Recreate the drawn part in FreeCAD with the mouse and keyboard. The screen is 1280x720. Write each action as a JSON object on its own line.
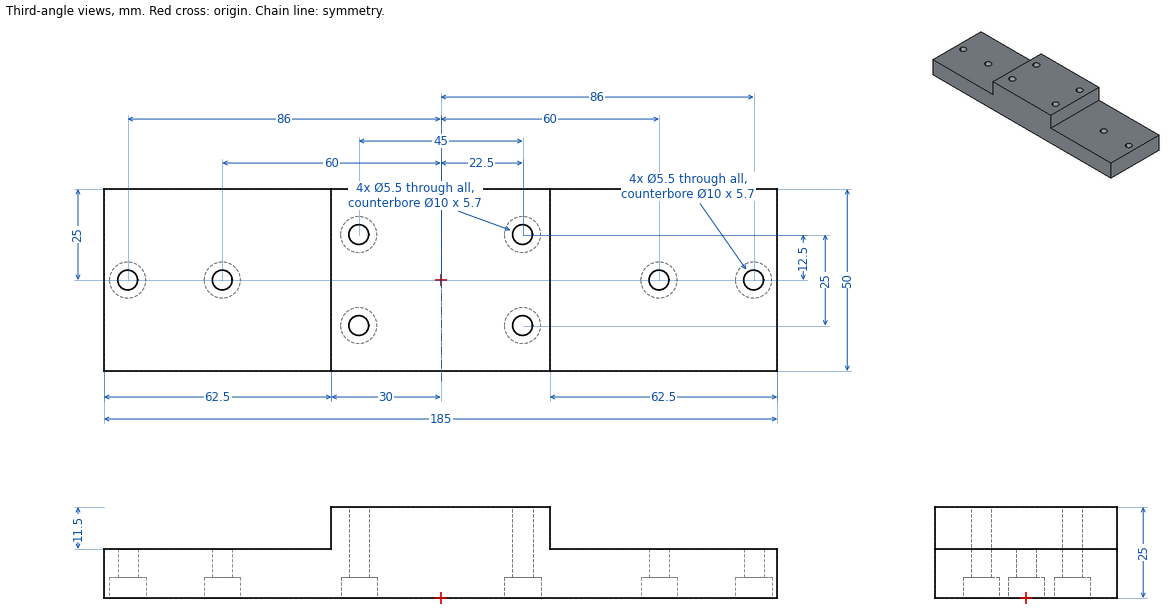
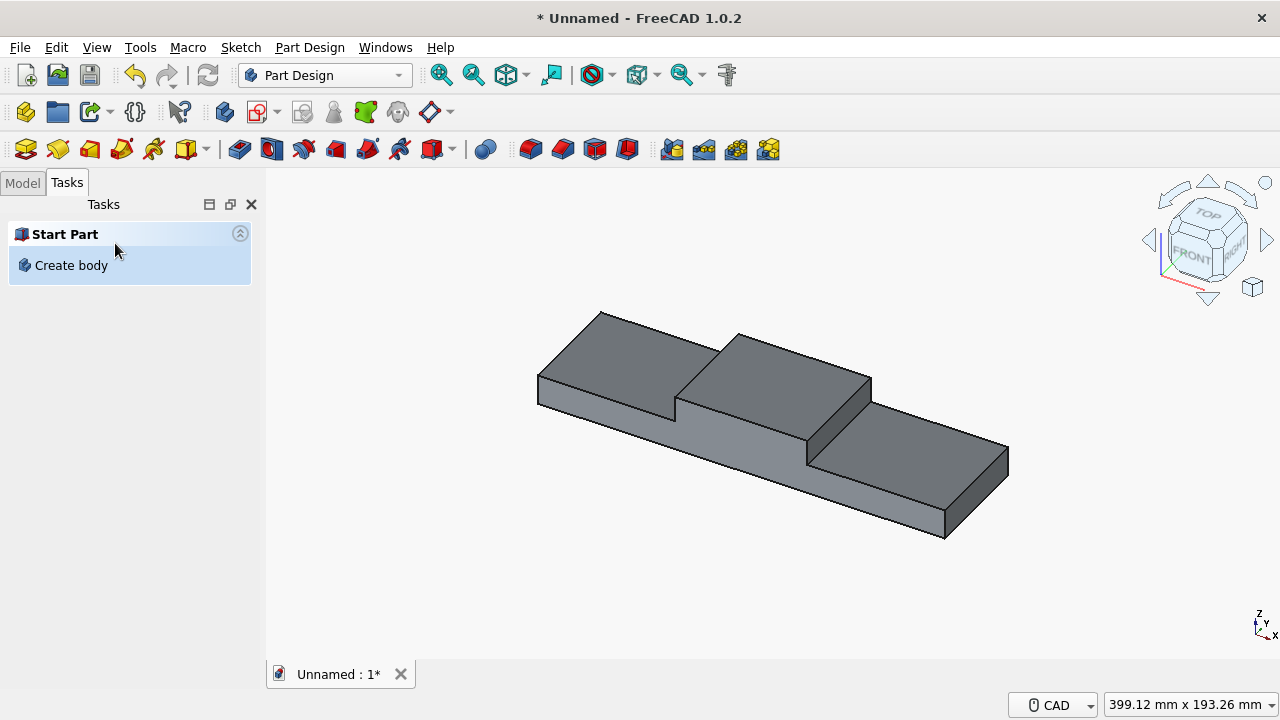
{"action": "key", "text": "5"}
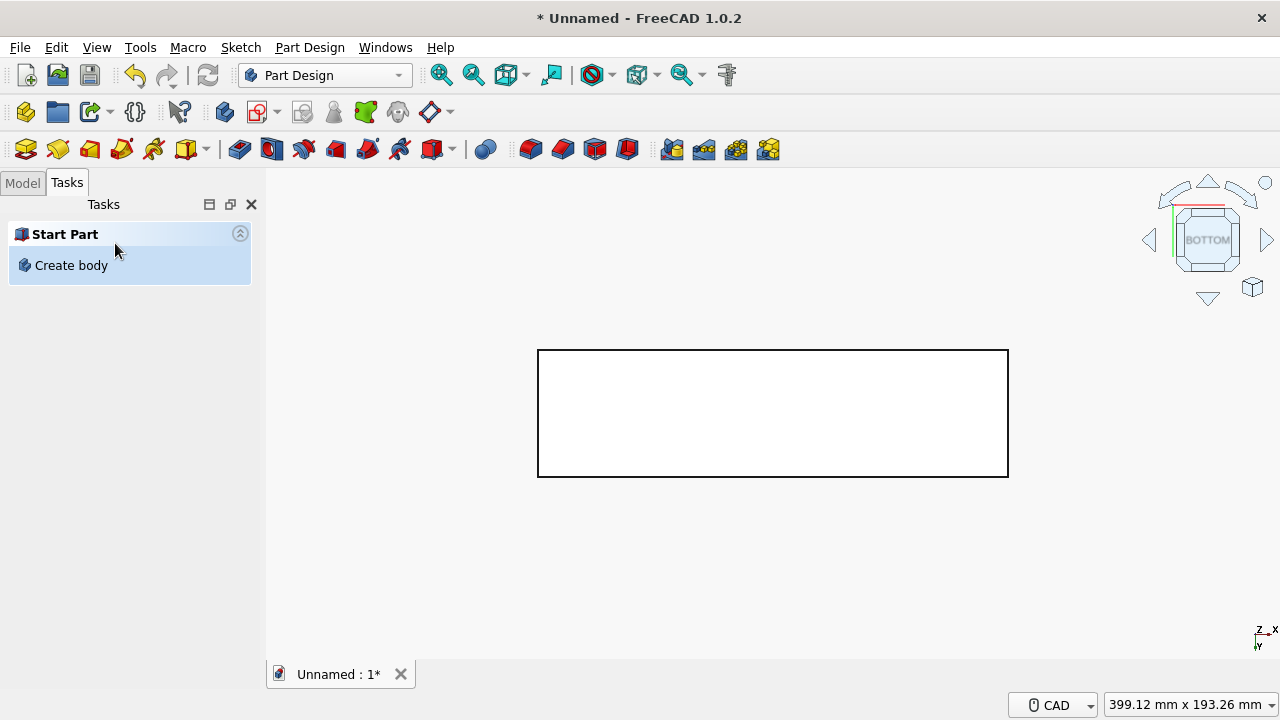
{"action": "left_click", "coordinate": [907, 412]}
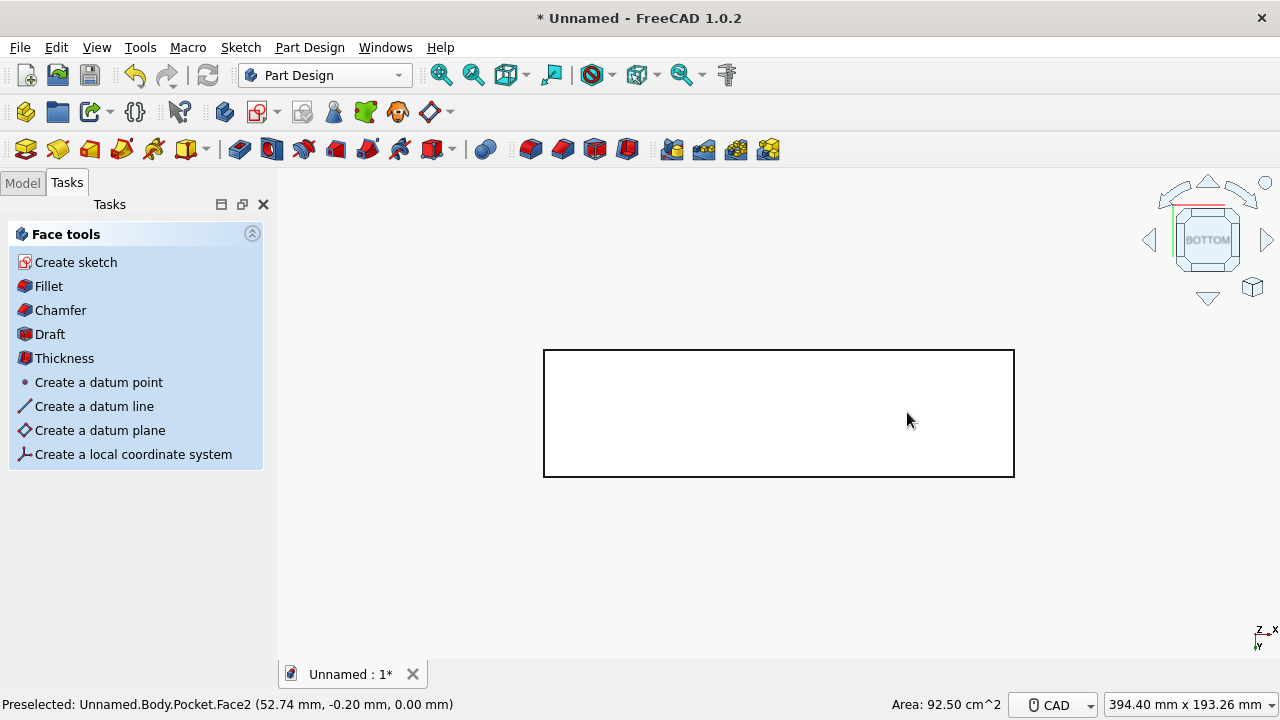
{"action": "left_click", "coordinate": [258, 112]}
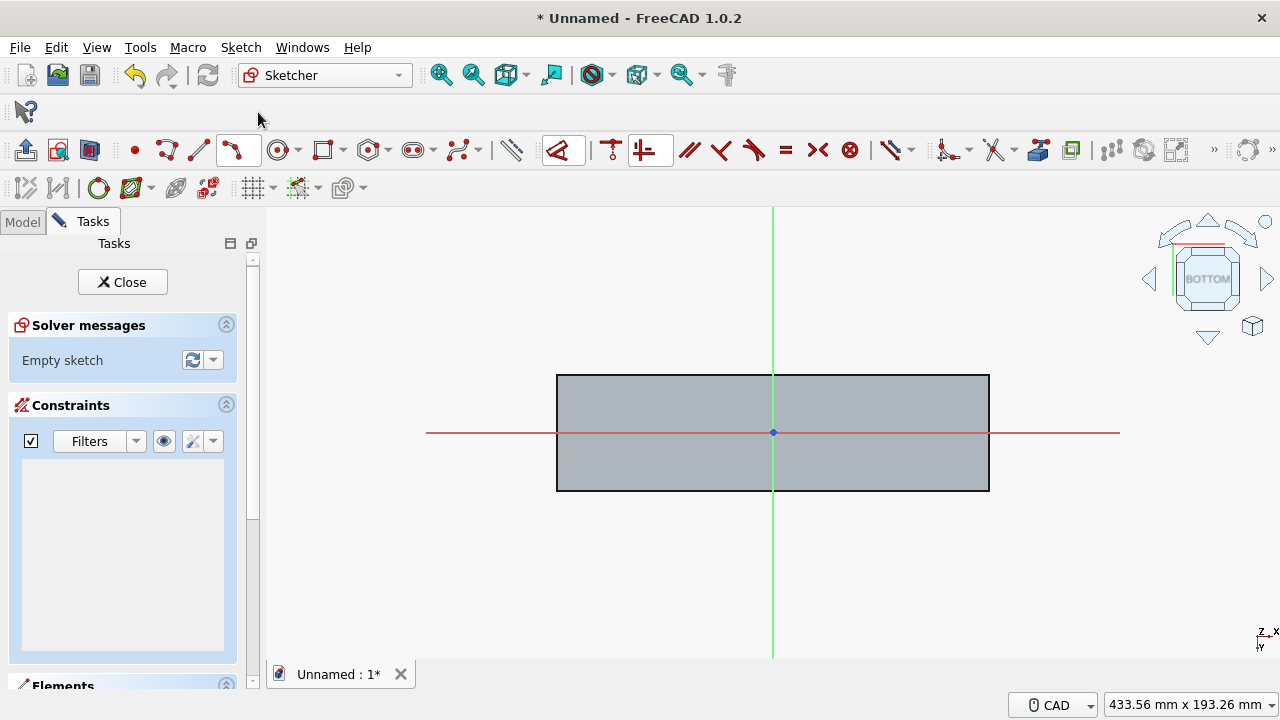
{"action": "scroll", "coordinate": [912, 433], "scroll_direction": "up", "scroll_amount": 2}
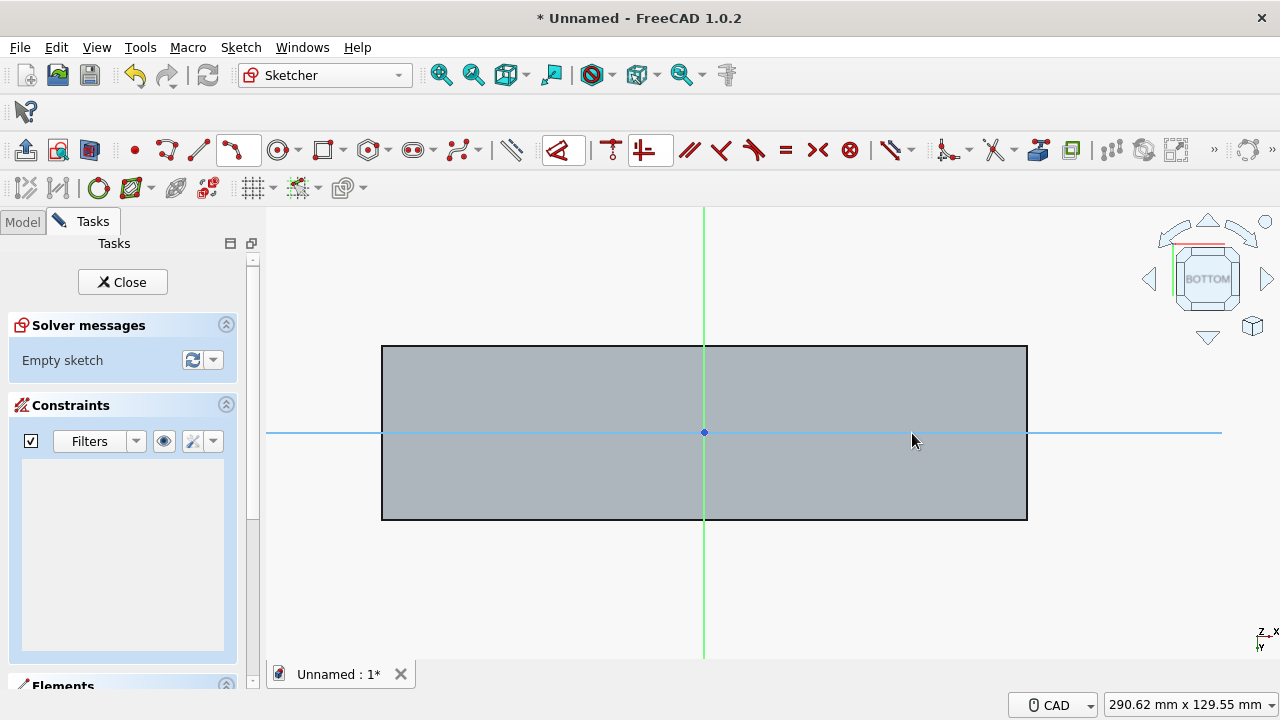
{"action": "left_click", "coordinate": [278, 150]}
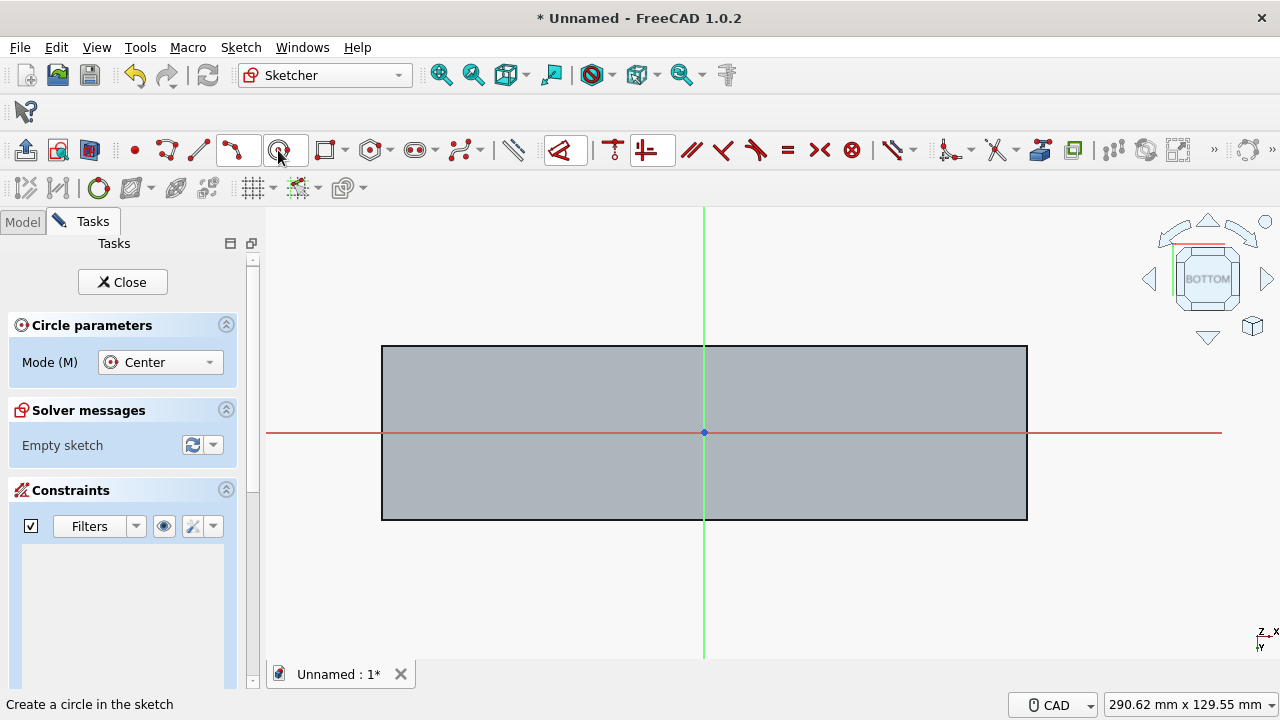
{"action": "scroll", "coordinate": [1004, 433], "scroll_direction": "up", "scroll_amount": 5}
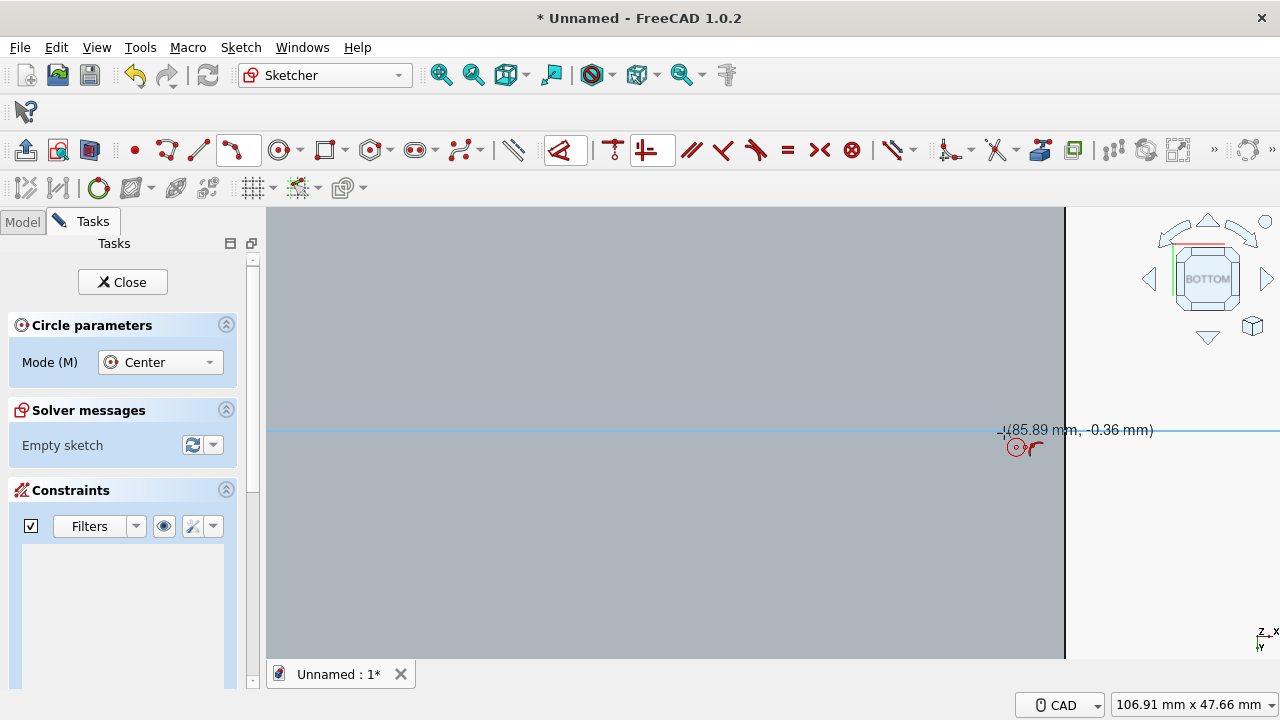
{"action": "left_click", "coordinate": [1004, 431]}
{"action": "mouse_move", "coordinate": [1022, 413]}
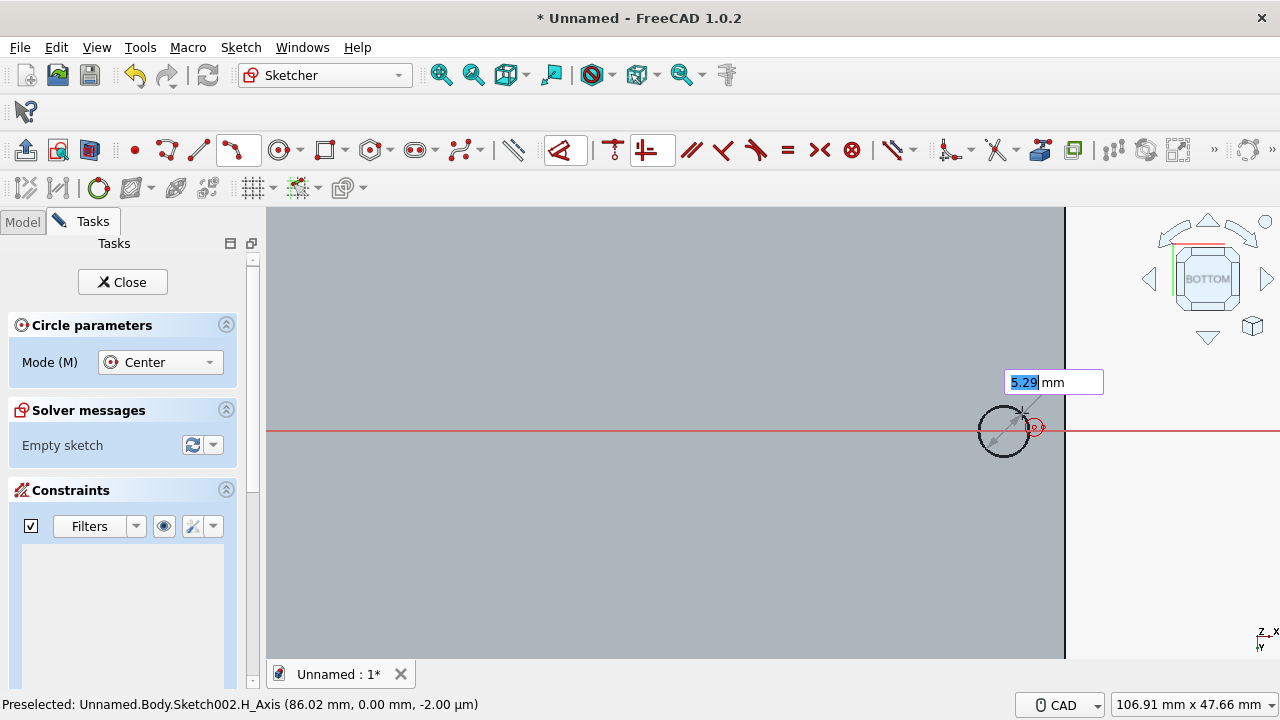
{"action": "type", "text": "5.5"}
{"action": "key", "text": "Return"}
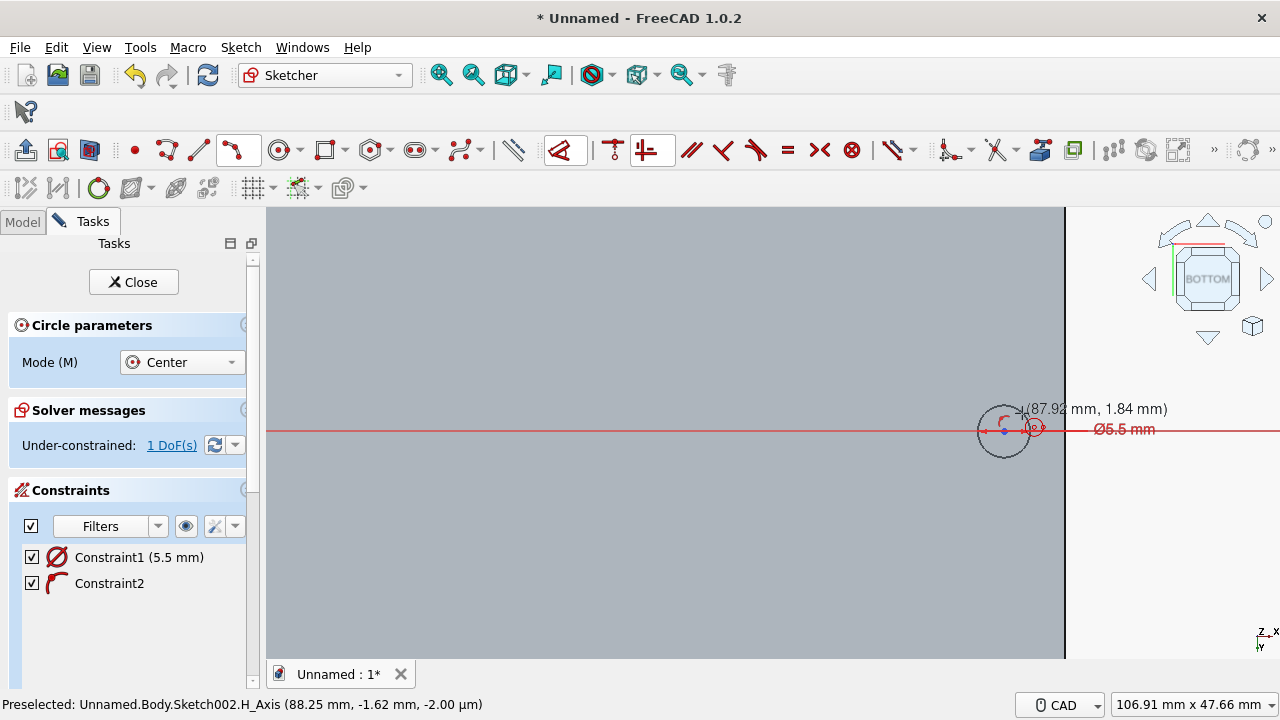
{"action": "left_click", "coordinate": [757, 431]}
{"action": "mouse_move", "coordinate": [776, 413]}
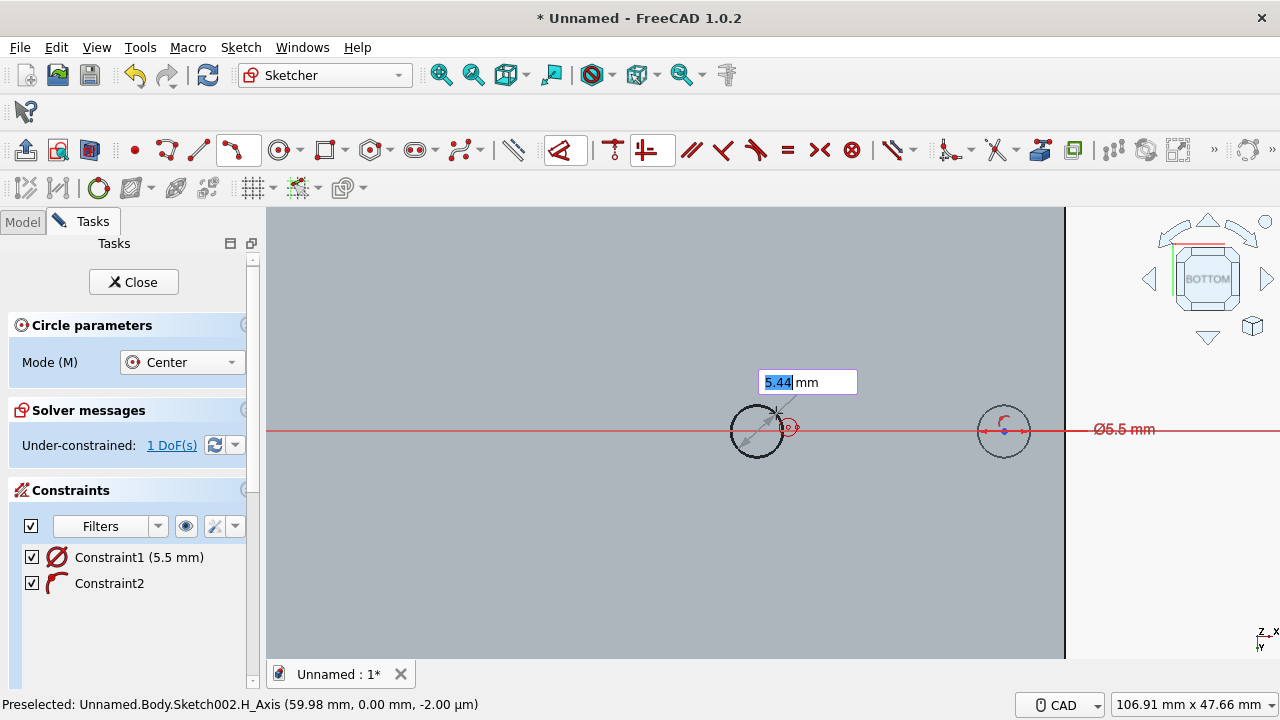
{"action": "type", "text": "5.5"}
{"action": "key", "text": "Return"}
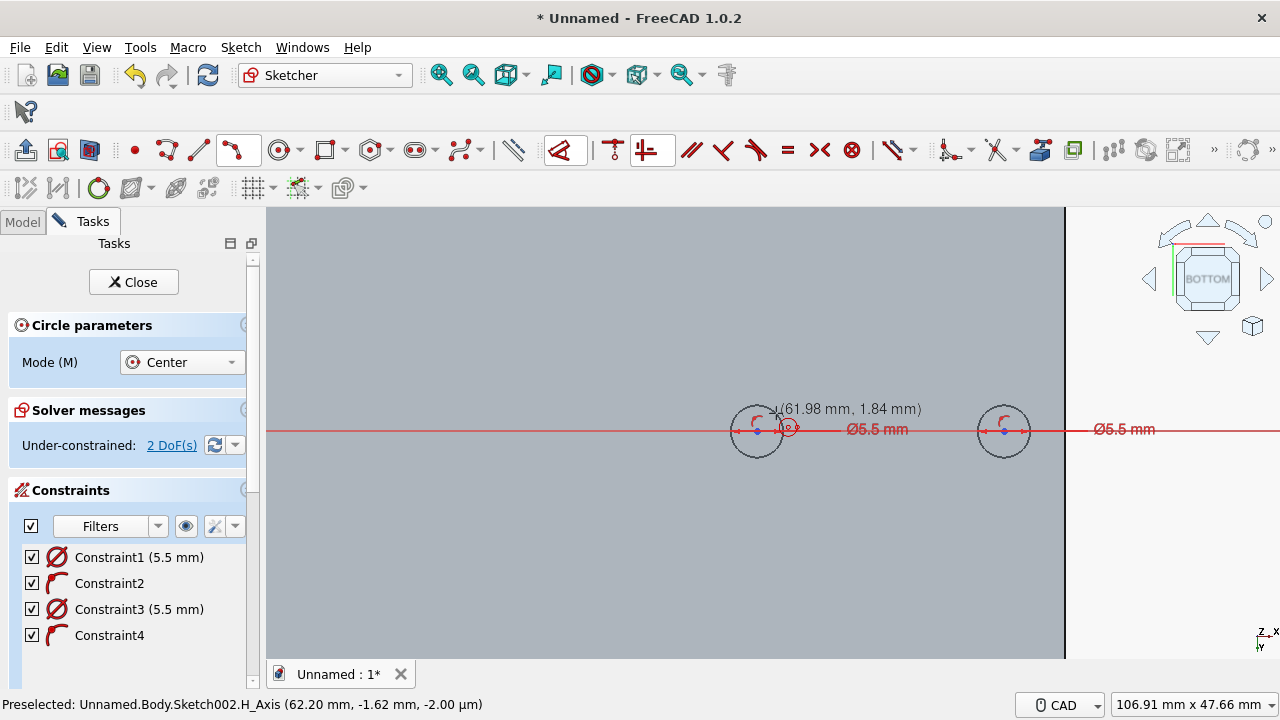
{"action": "scroll", "coordinate": [1005, 434], "scroll_direction": "down", "scroll_amount": 5}